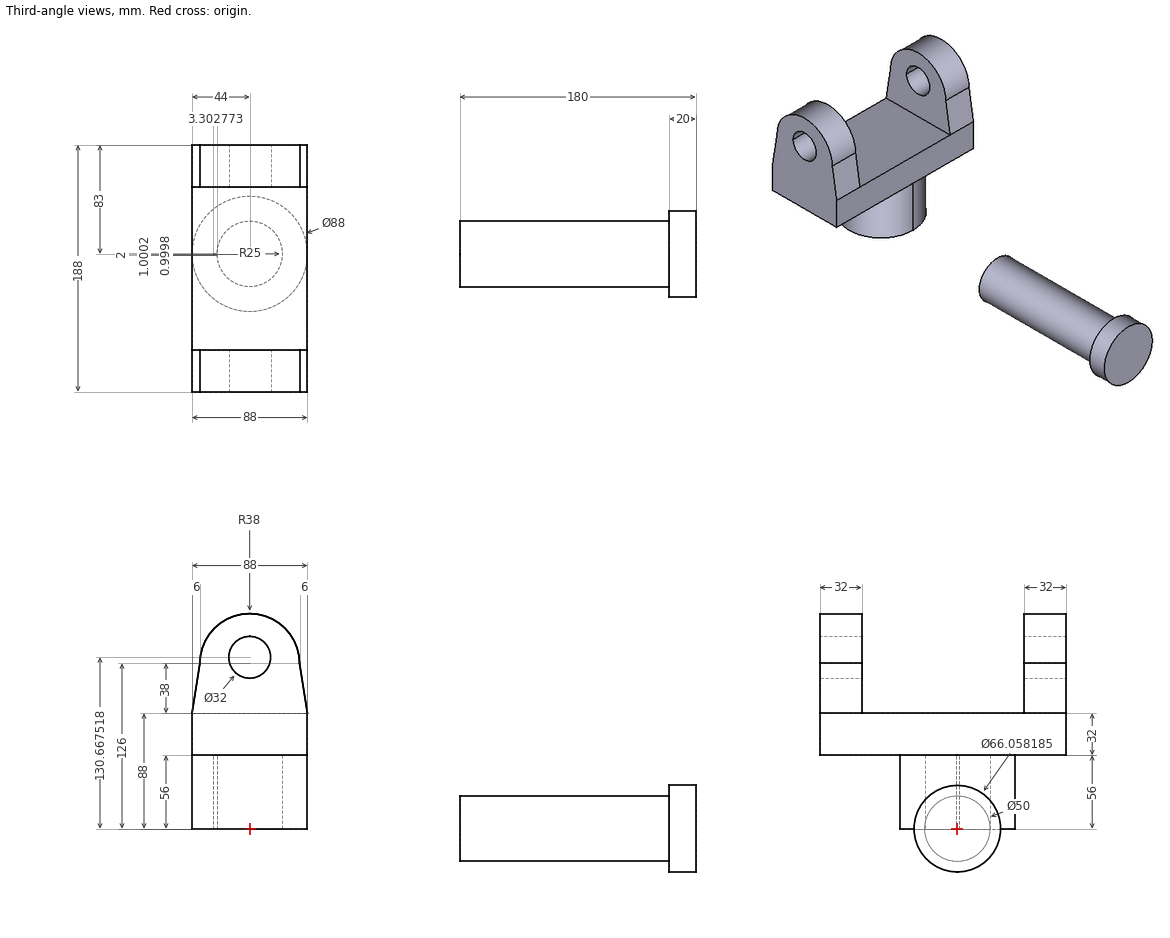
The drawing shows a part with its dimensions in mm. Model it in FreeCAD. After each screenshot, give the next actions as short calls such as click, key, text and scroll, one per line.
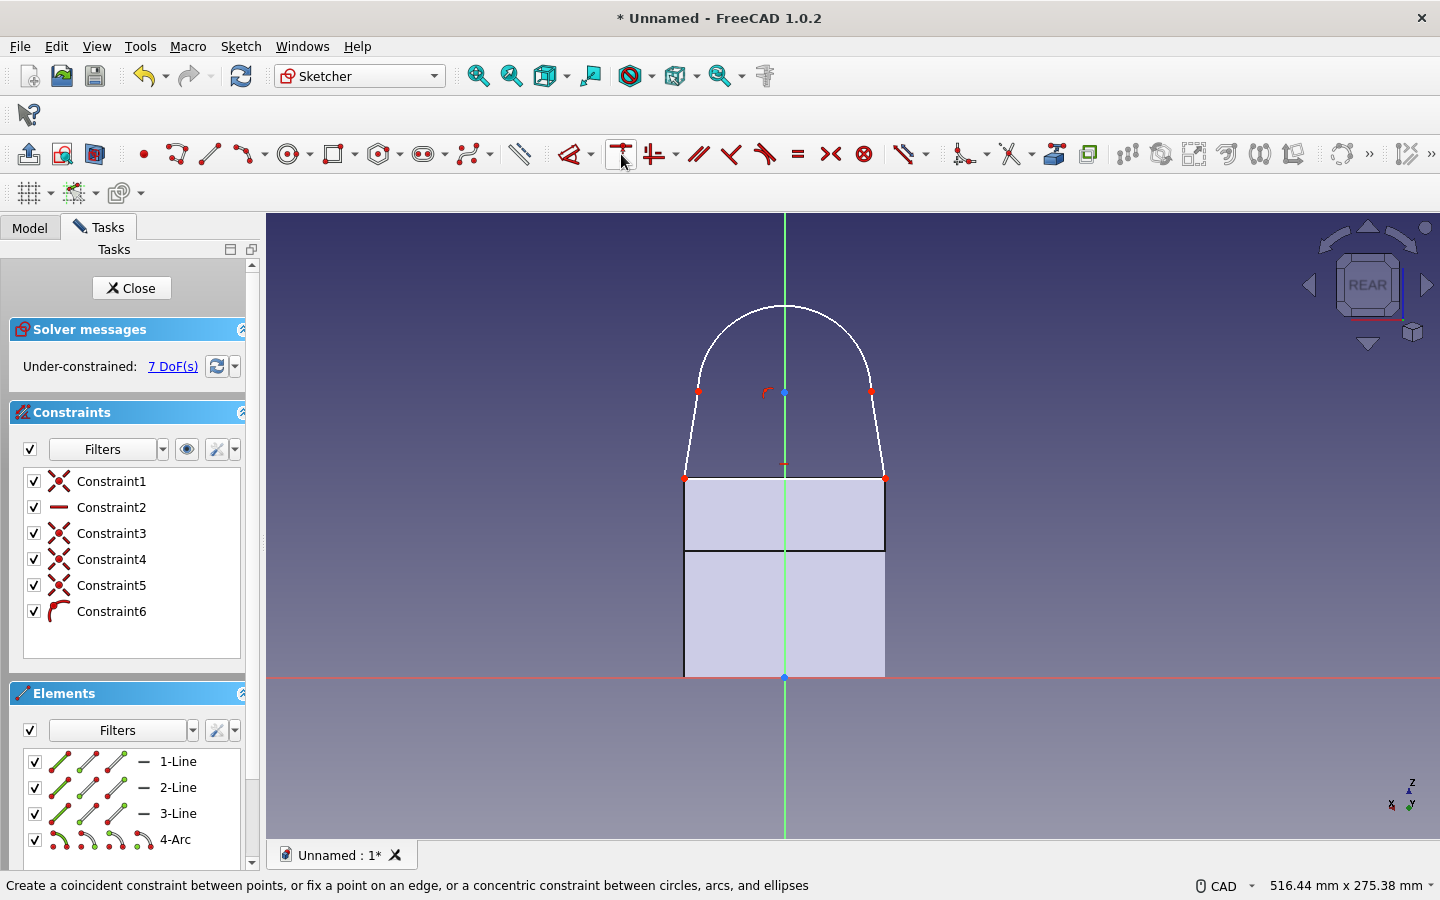
key(d)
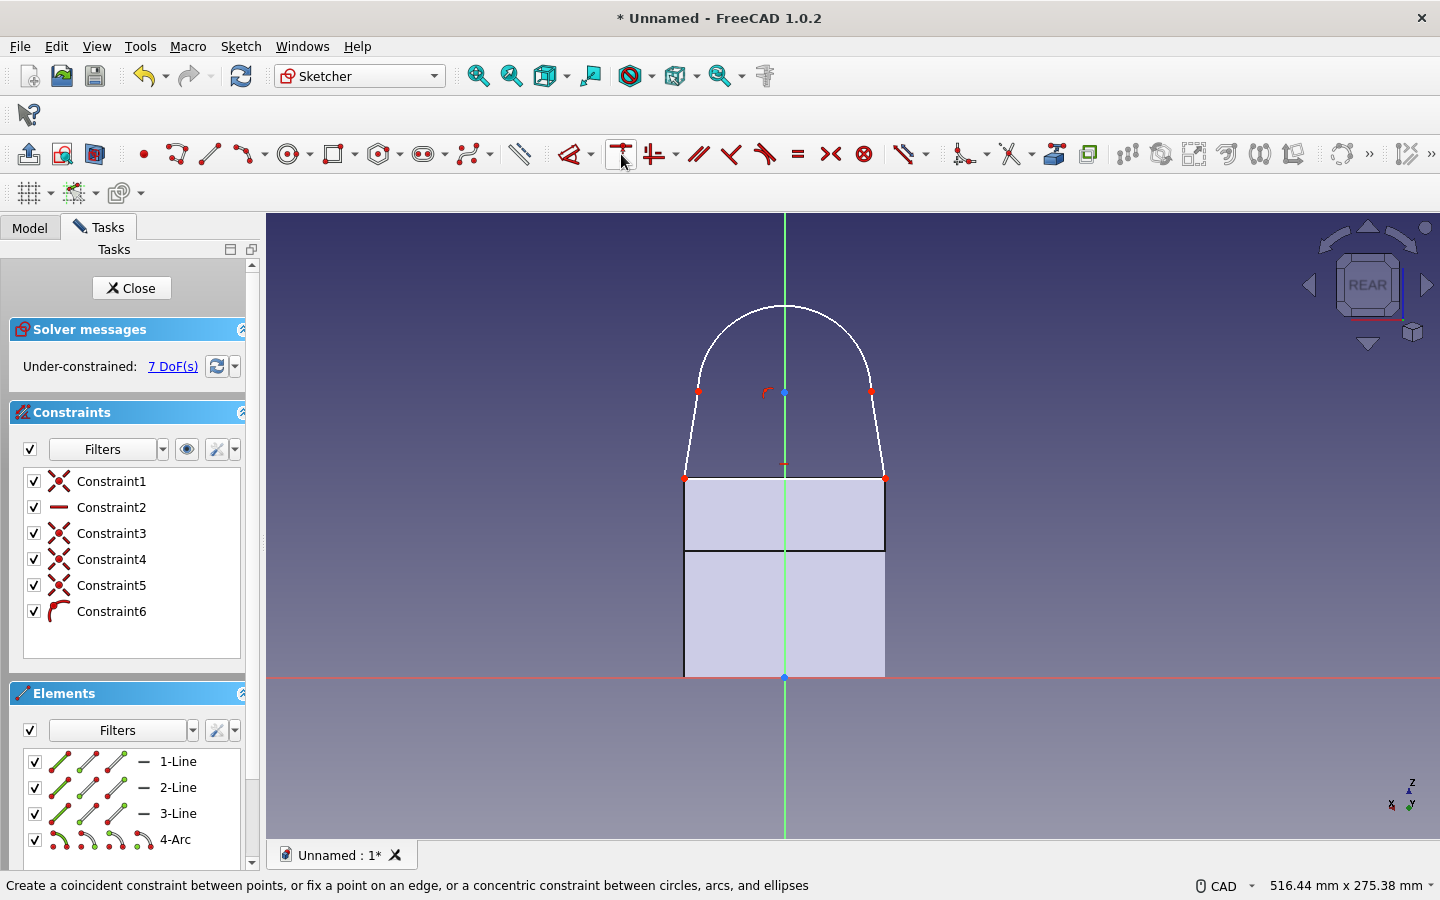
click(835, 322)
click(854, 296)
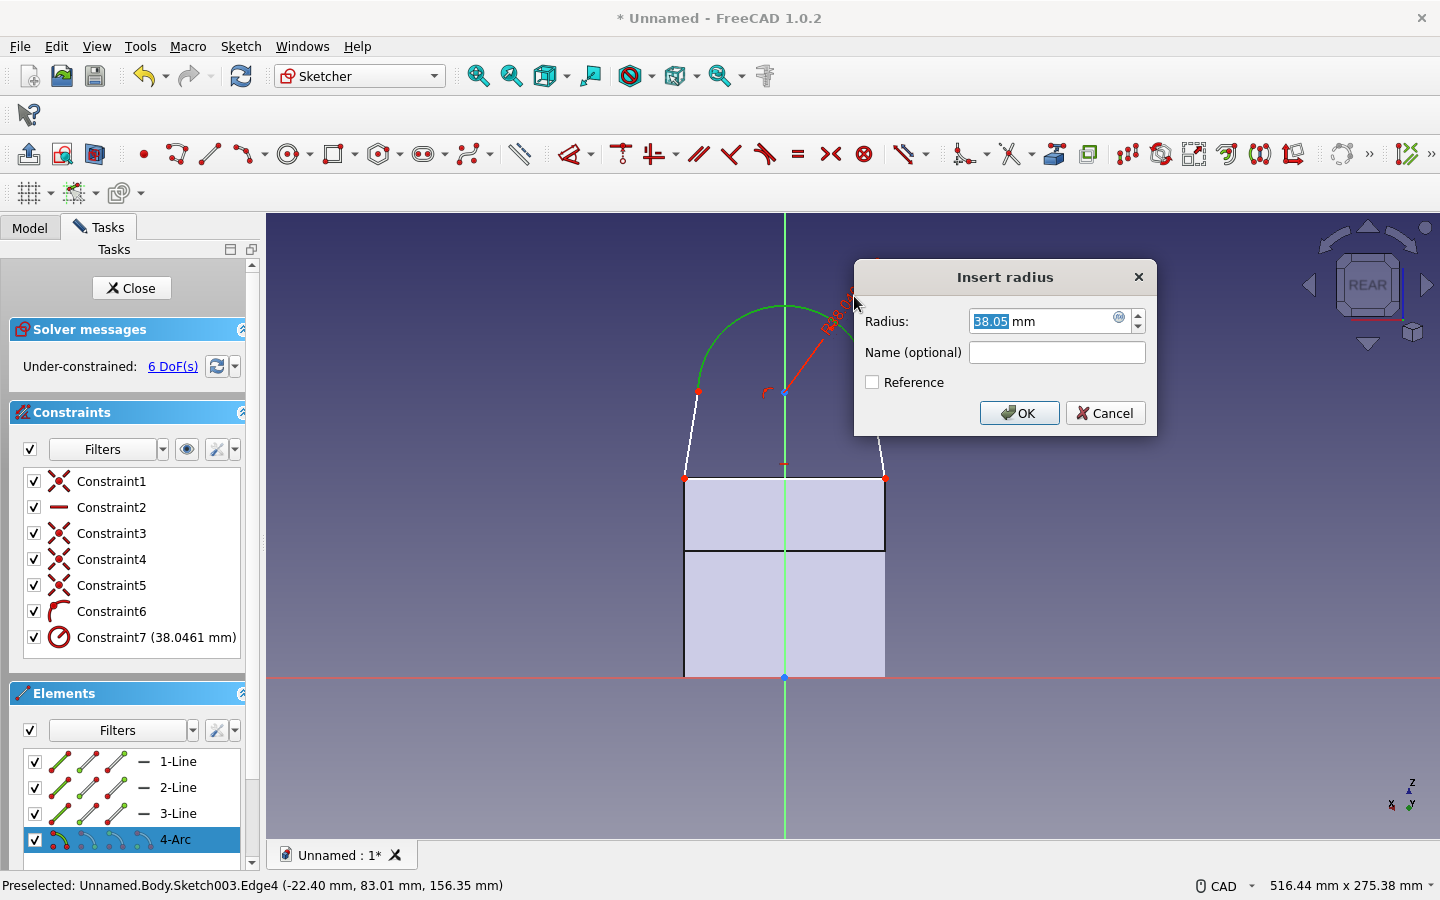
text(38)
key(Return)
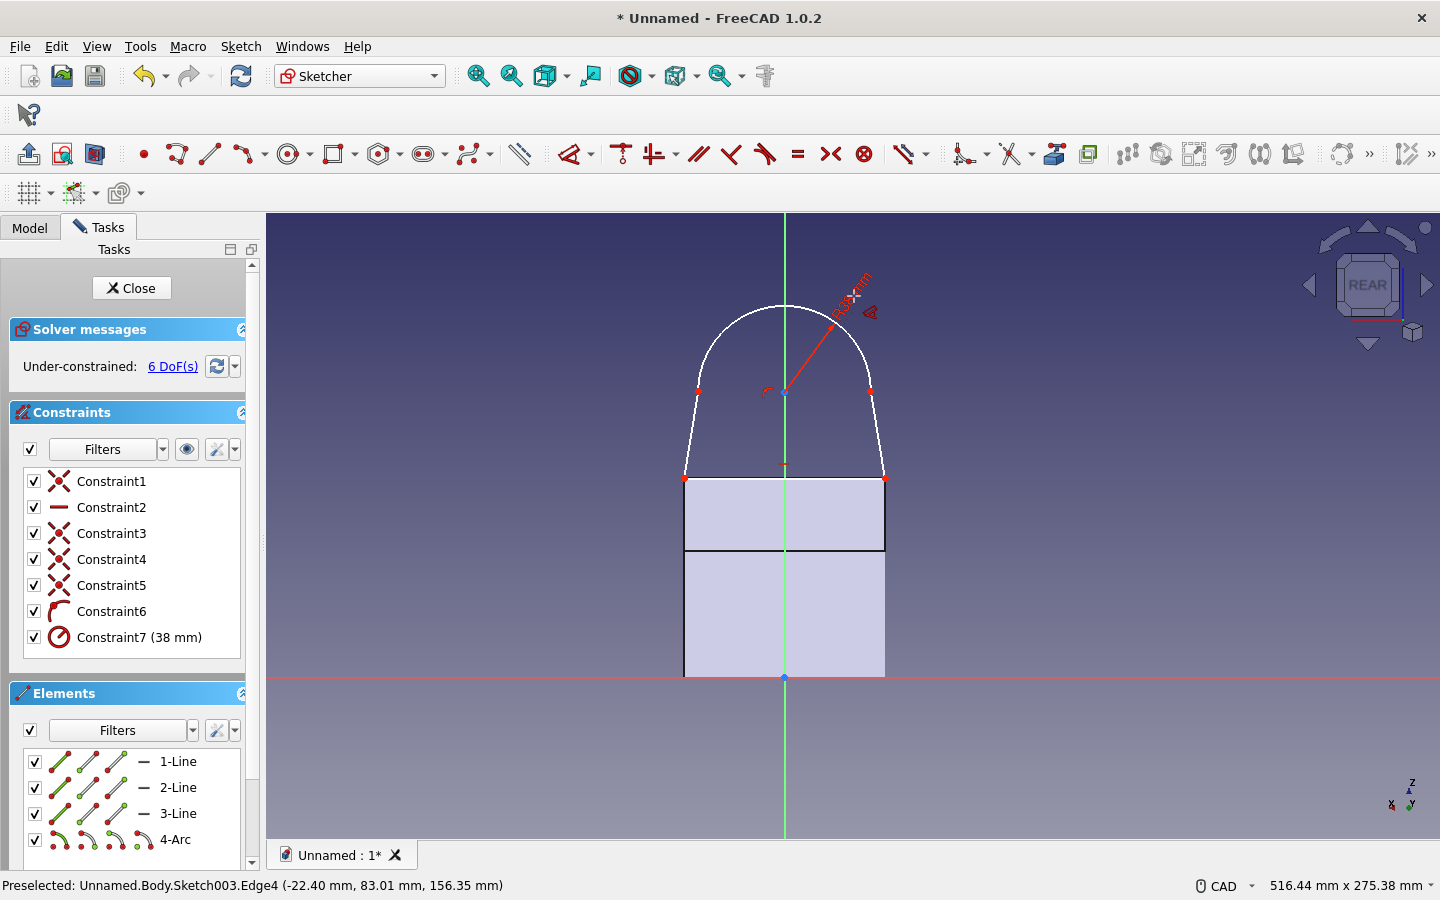
click(744, 479)
click(738, 445)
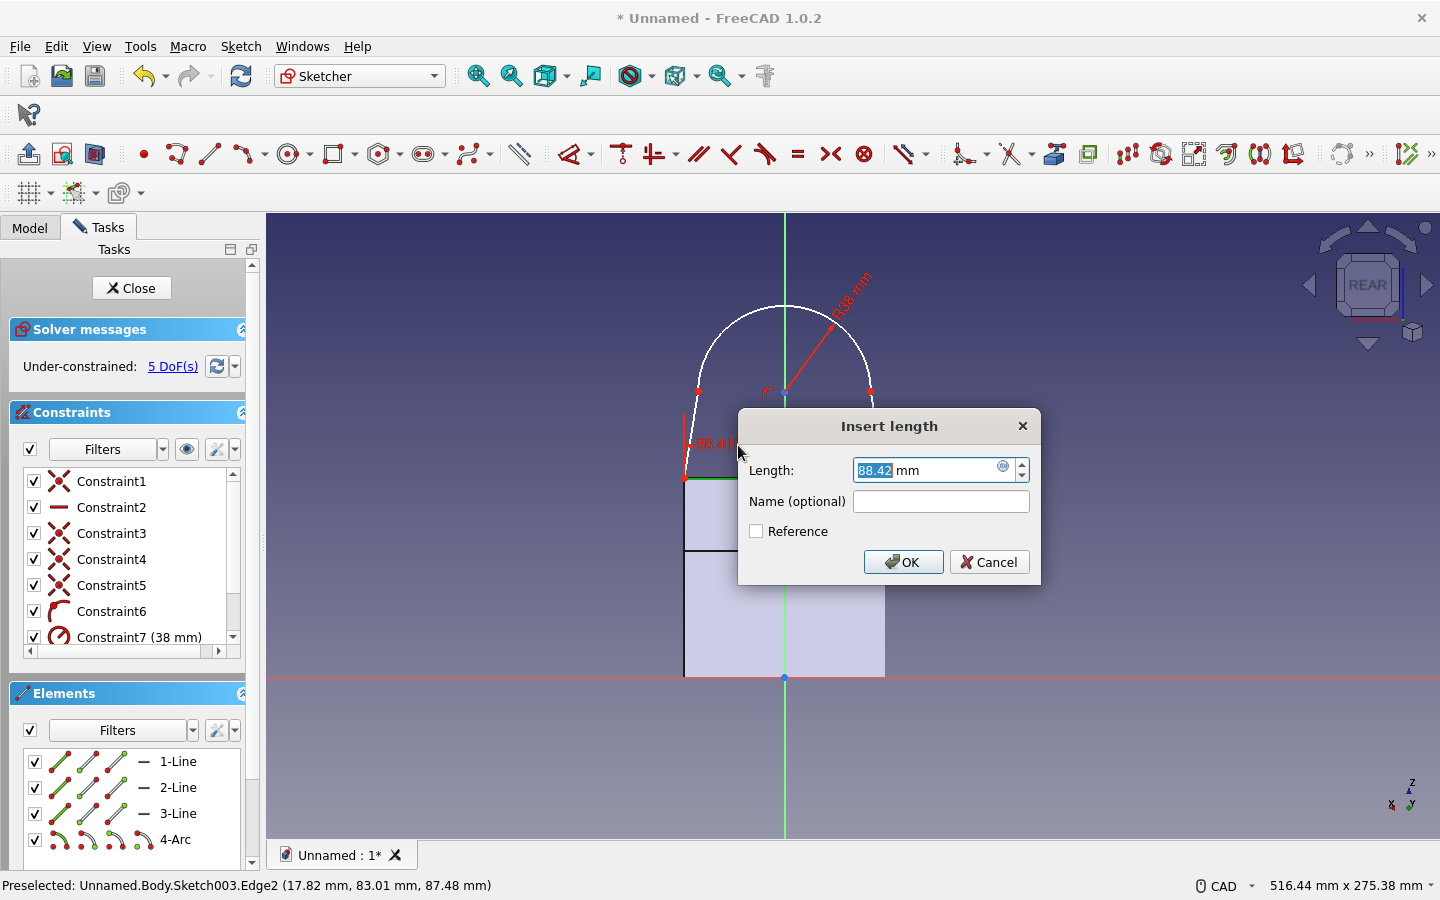
text(88)
key(Return)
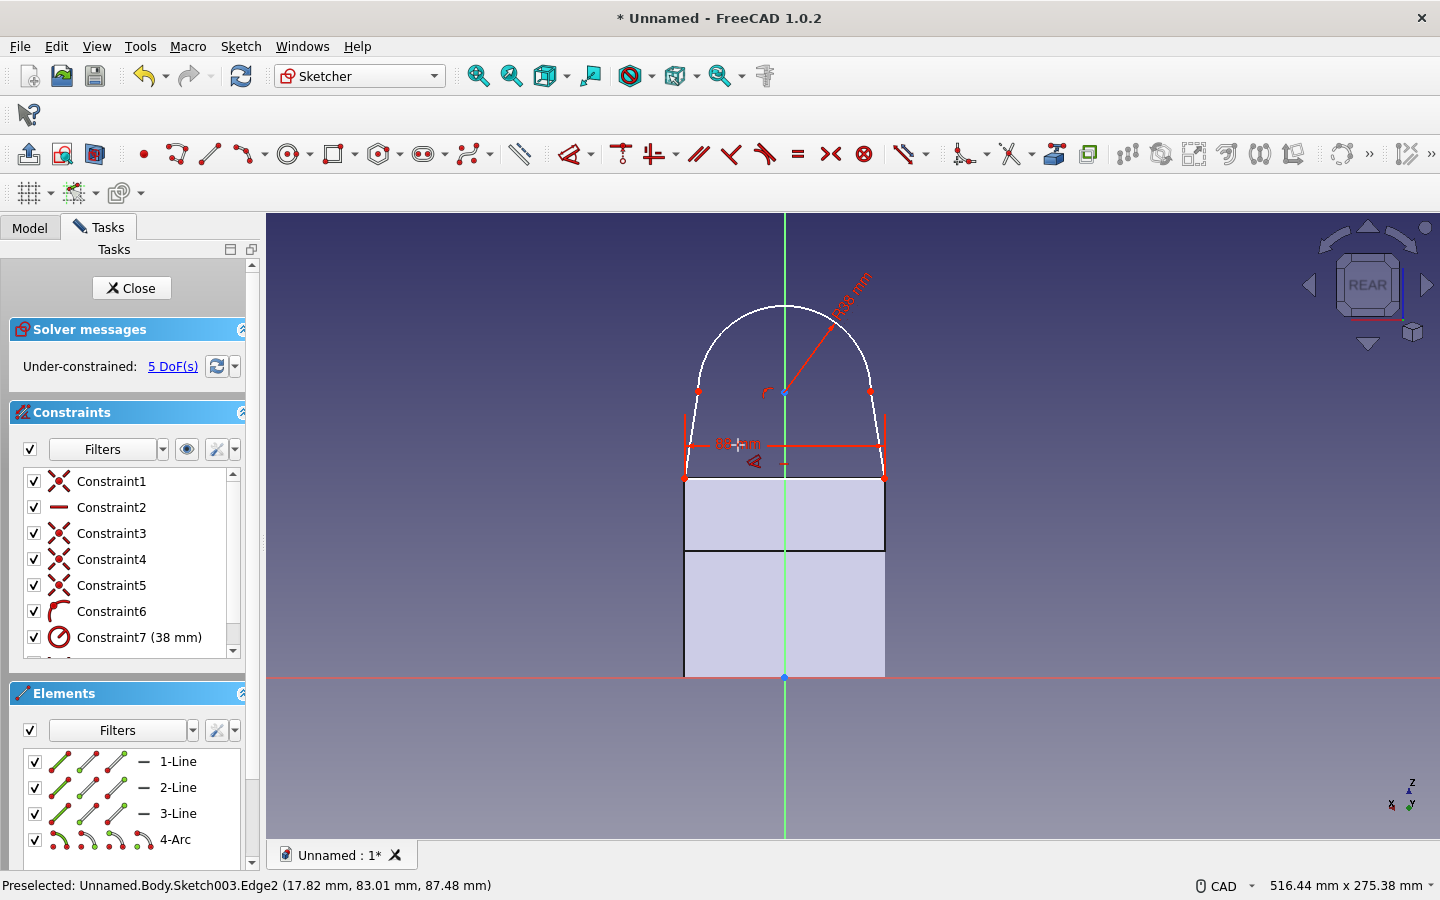
scroll(694, 418, up, 6)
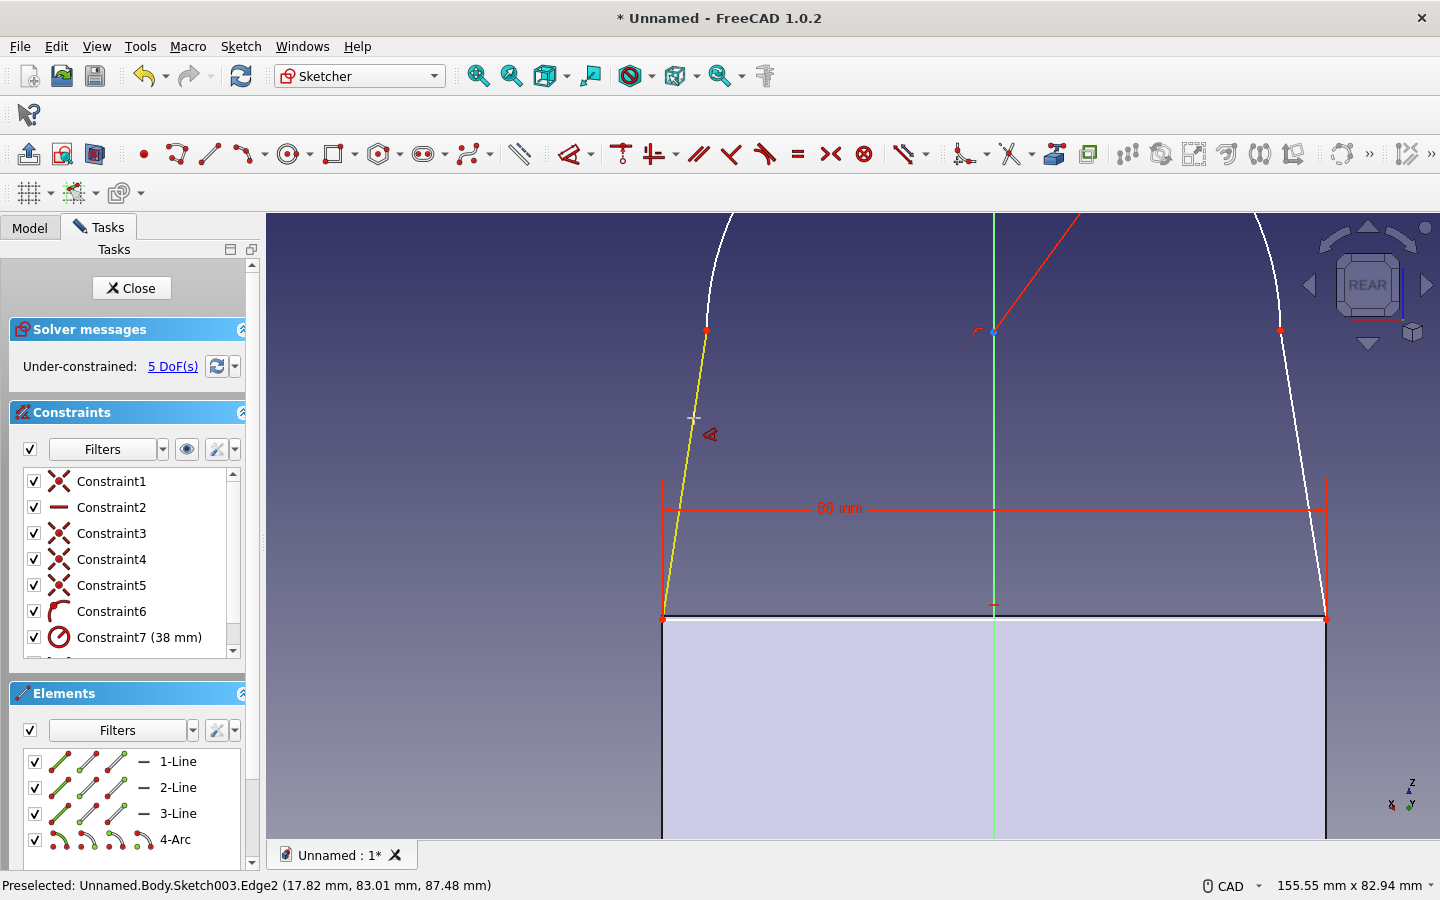
click(694, 418)
click(685, 297)